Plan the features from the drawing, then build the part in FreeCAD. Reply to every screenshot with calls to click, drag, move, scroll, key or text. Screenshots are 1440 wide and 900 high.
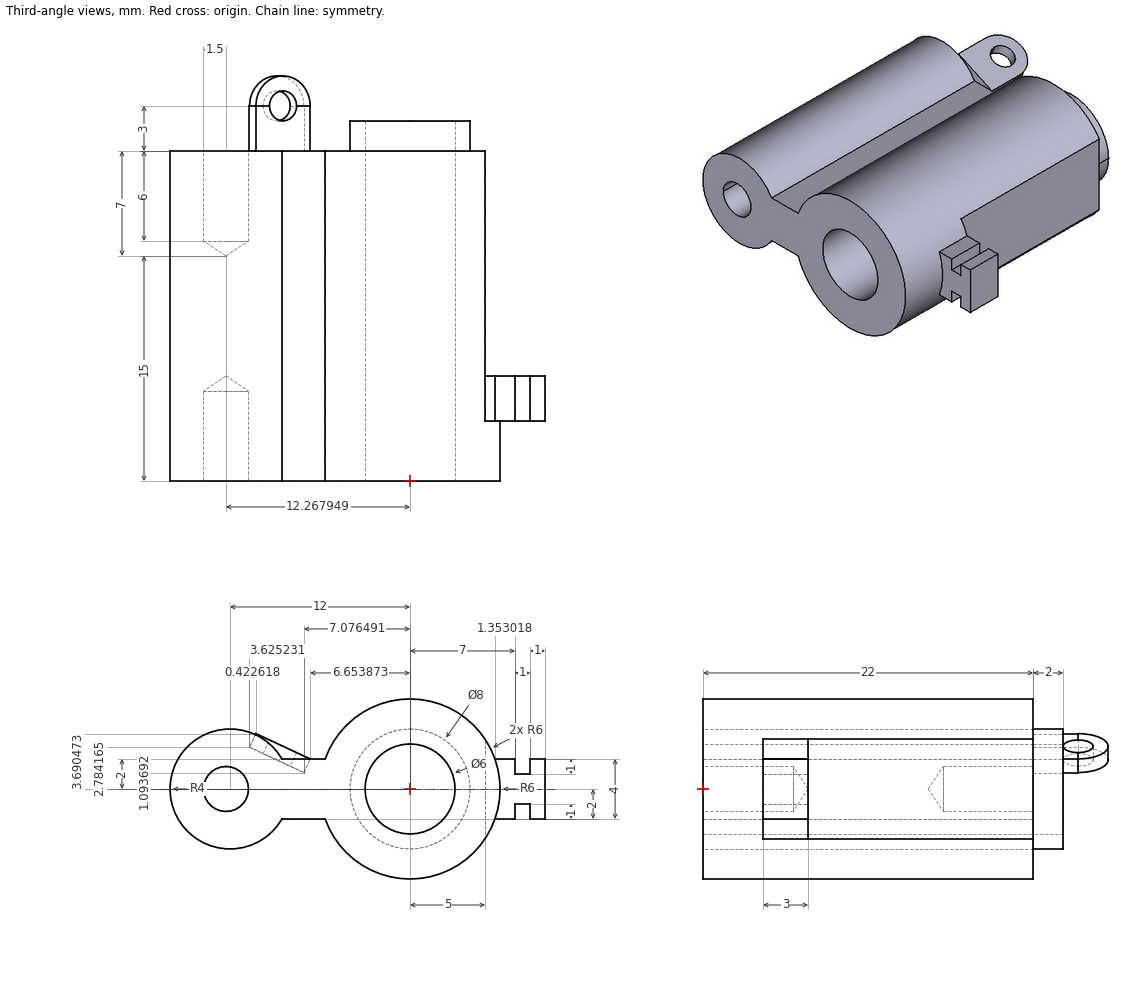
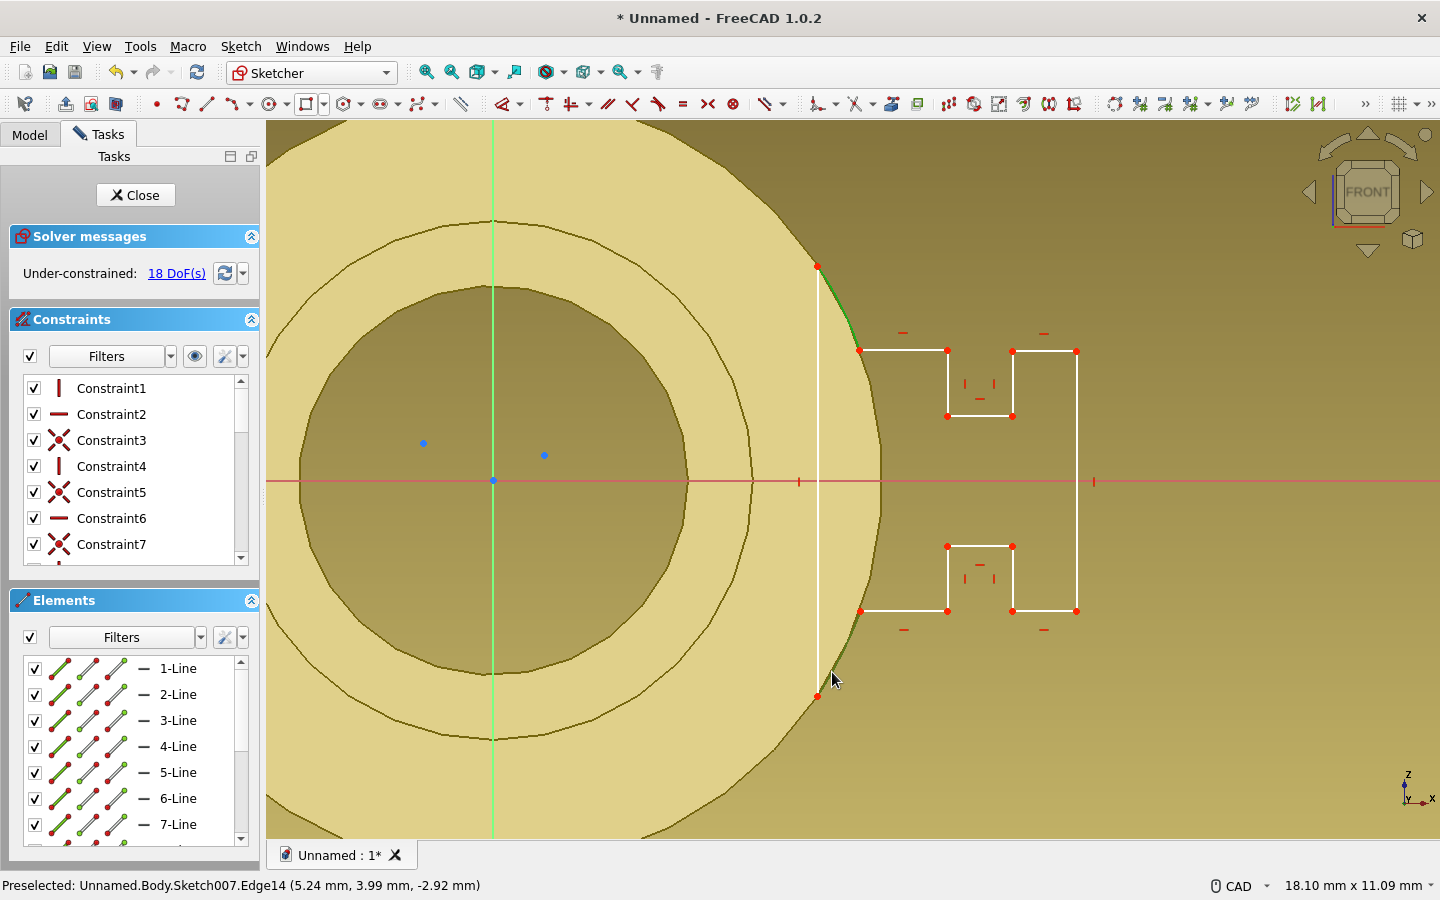
click(546, 104)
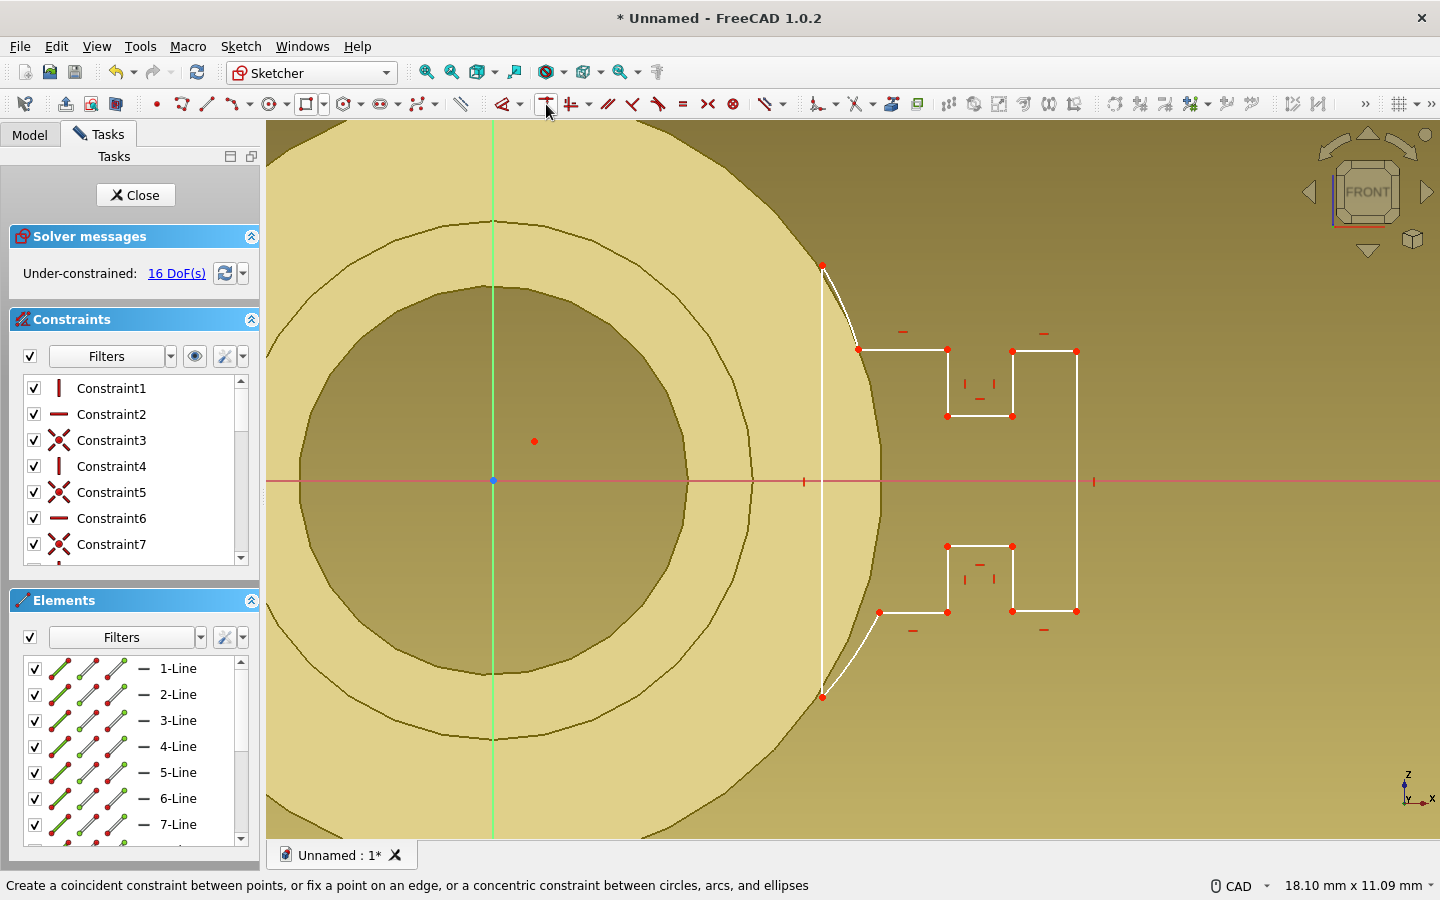
drag(483, 432, 545, 491)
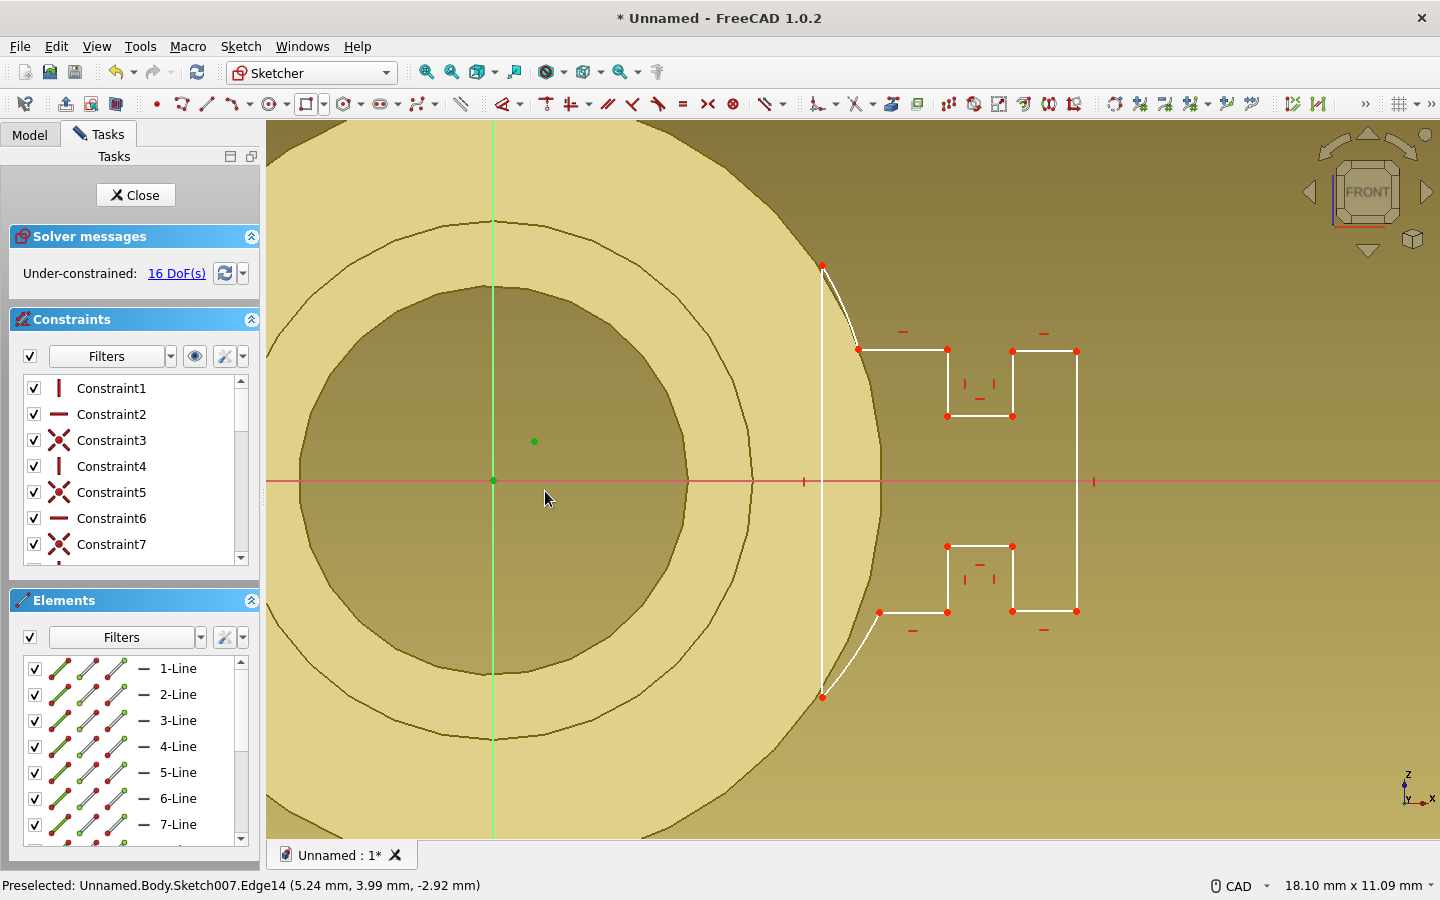
click(546, 104)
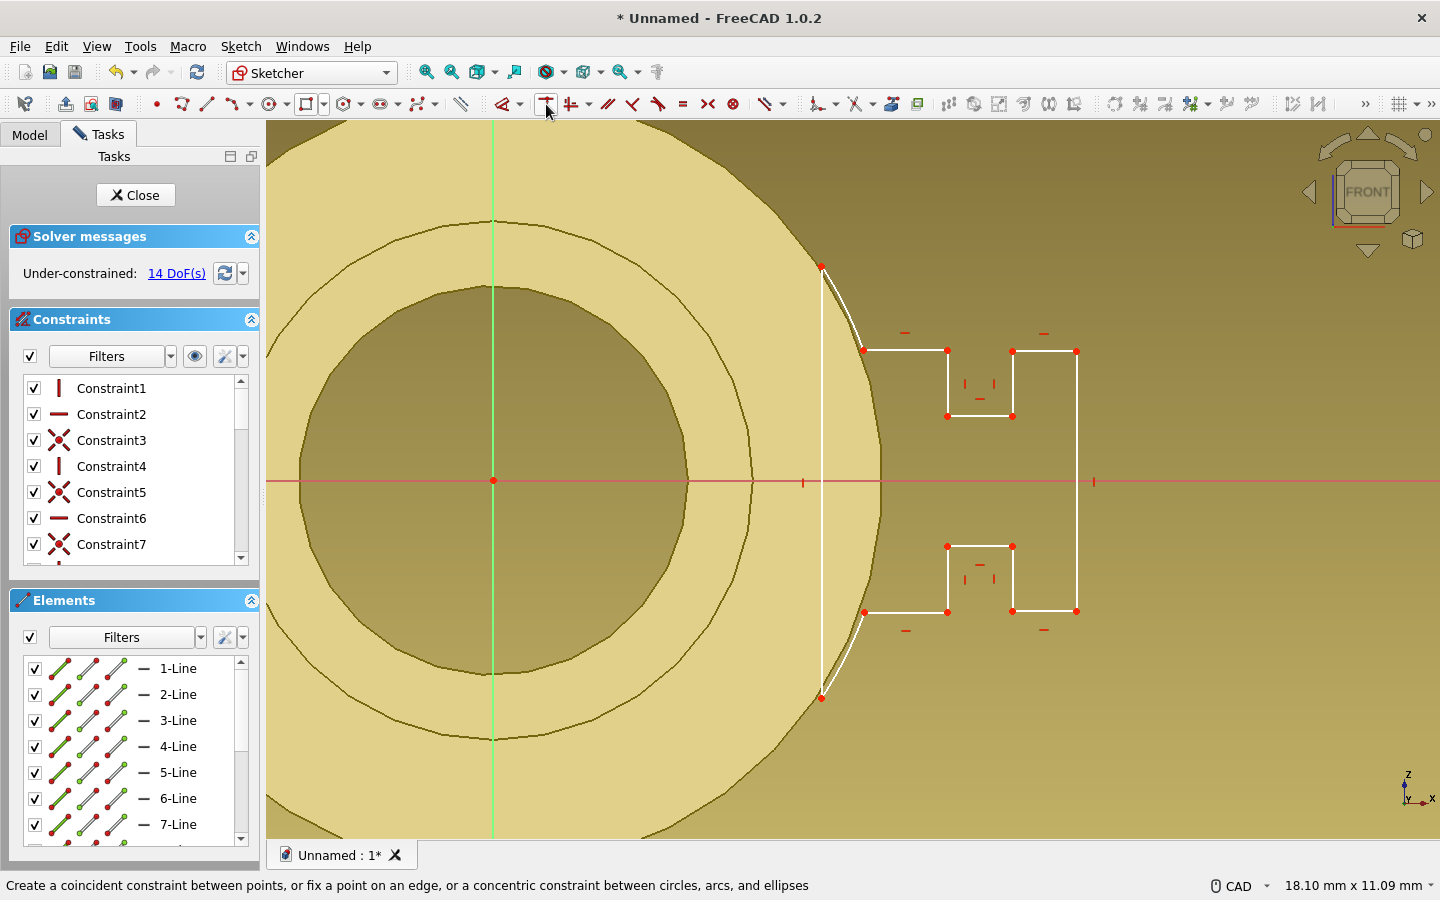
click(853, 324)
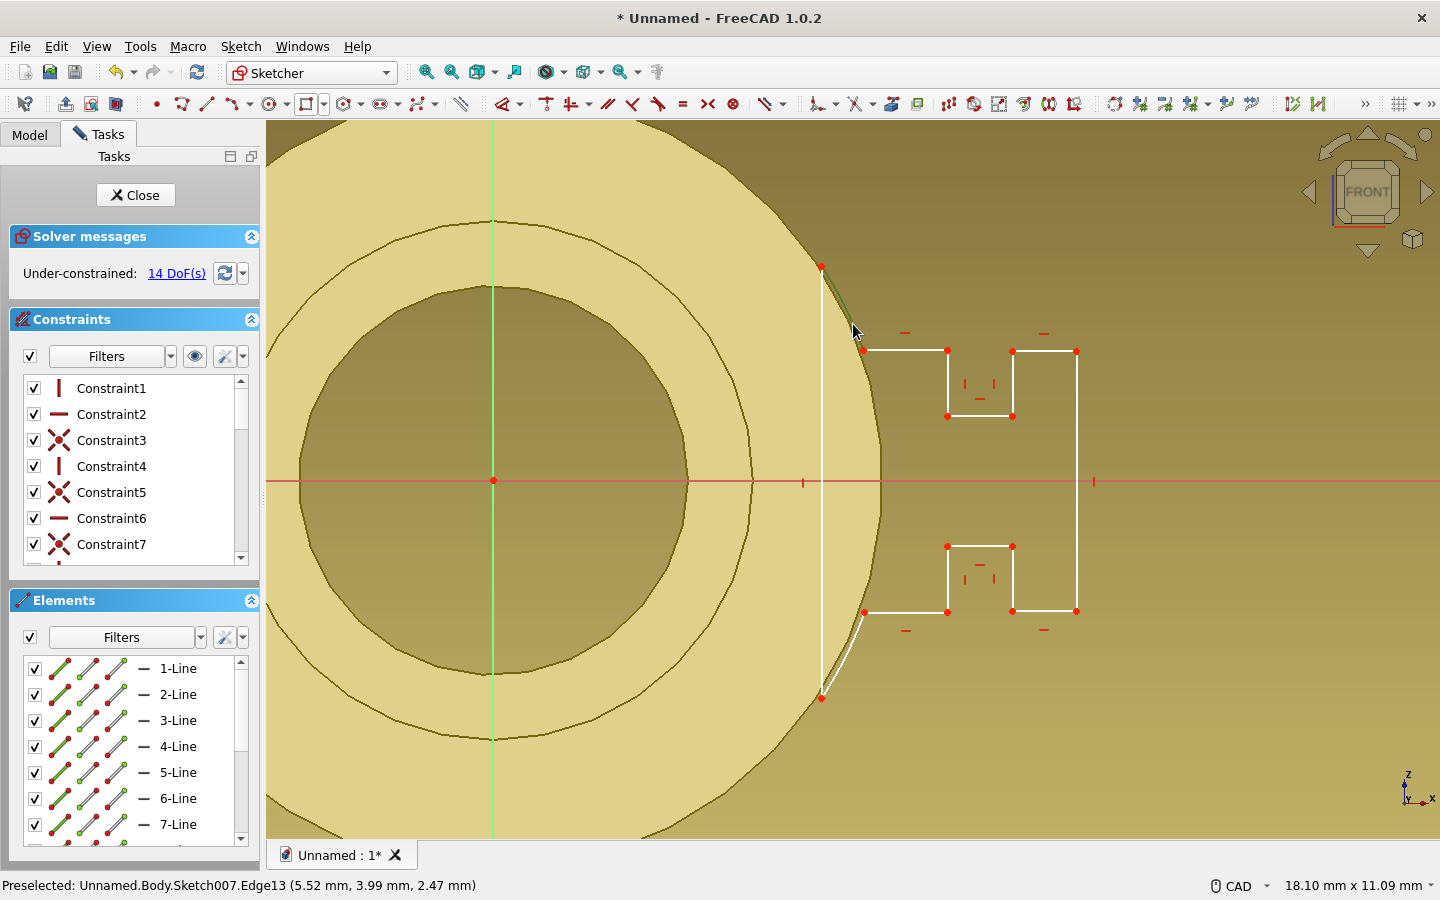
click(837, 674)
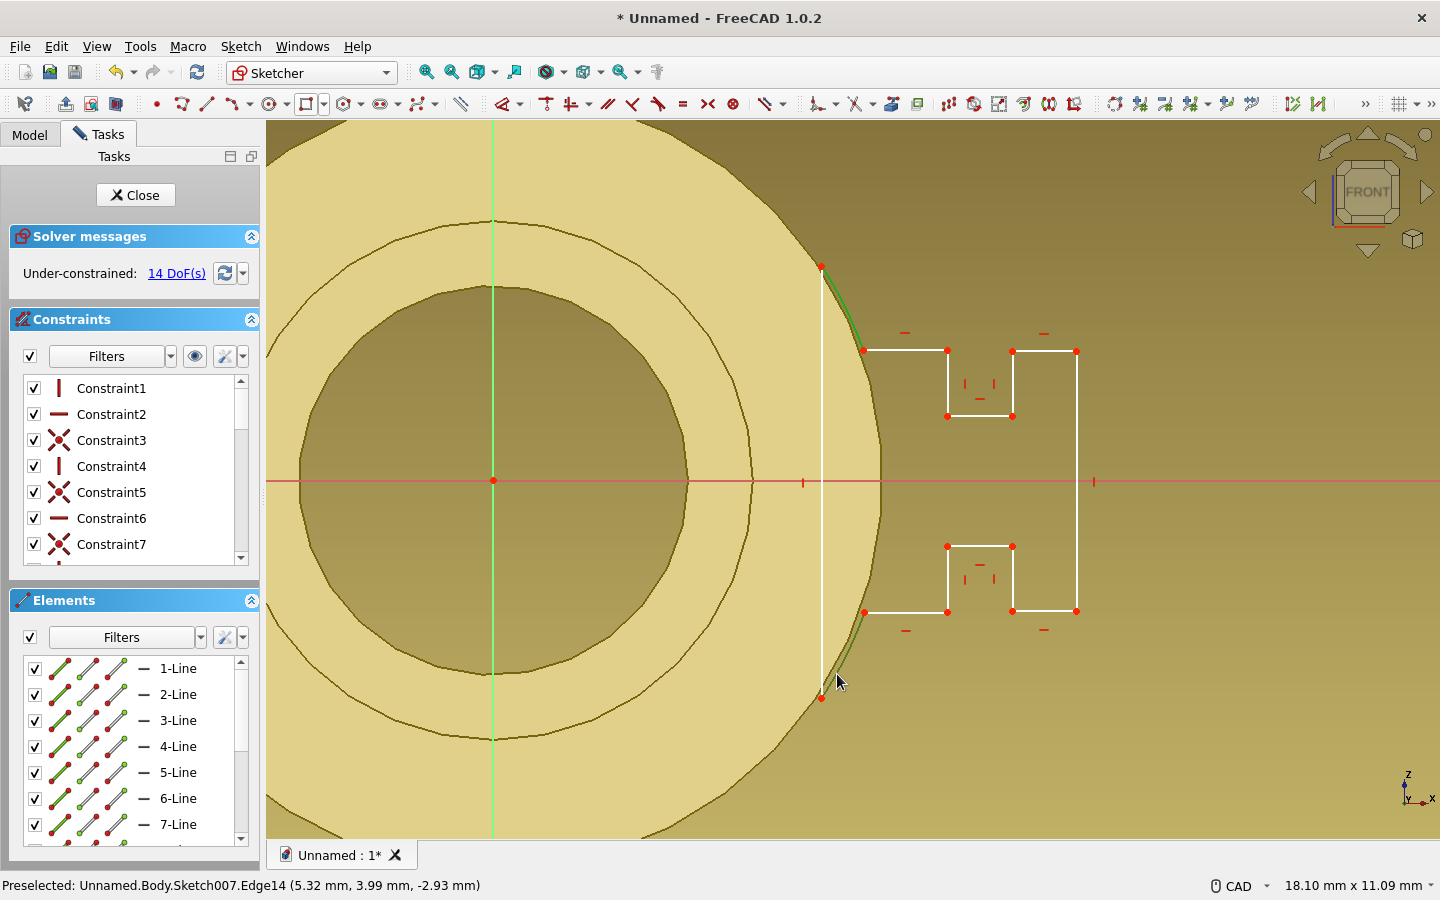
click(683, 104)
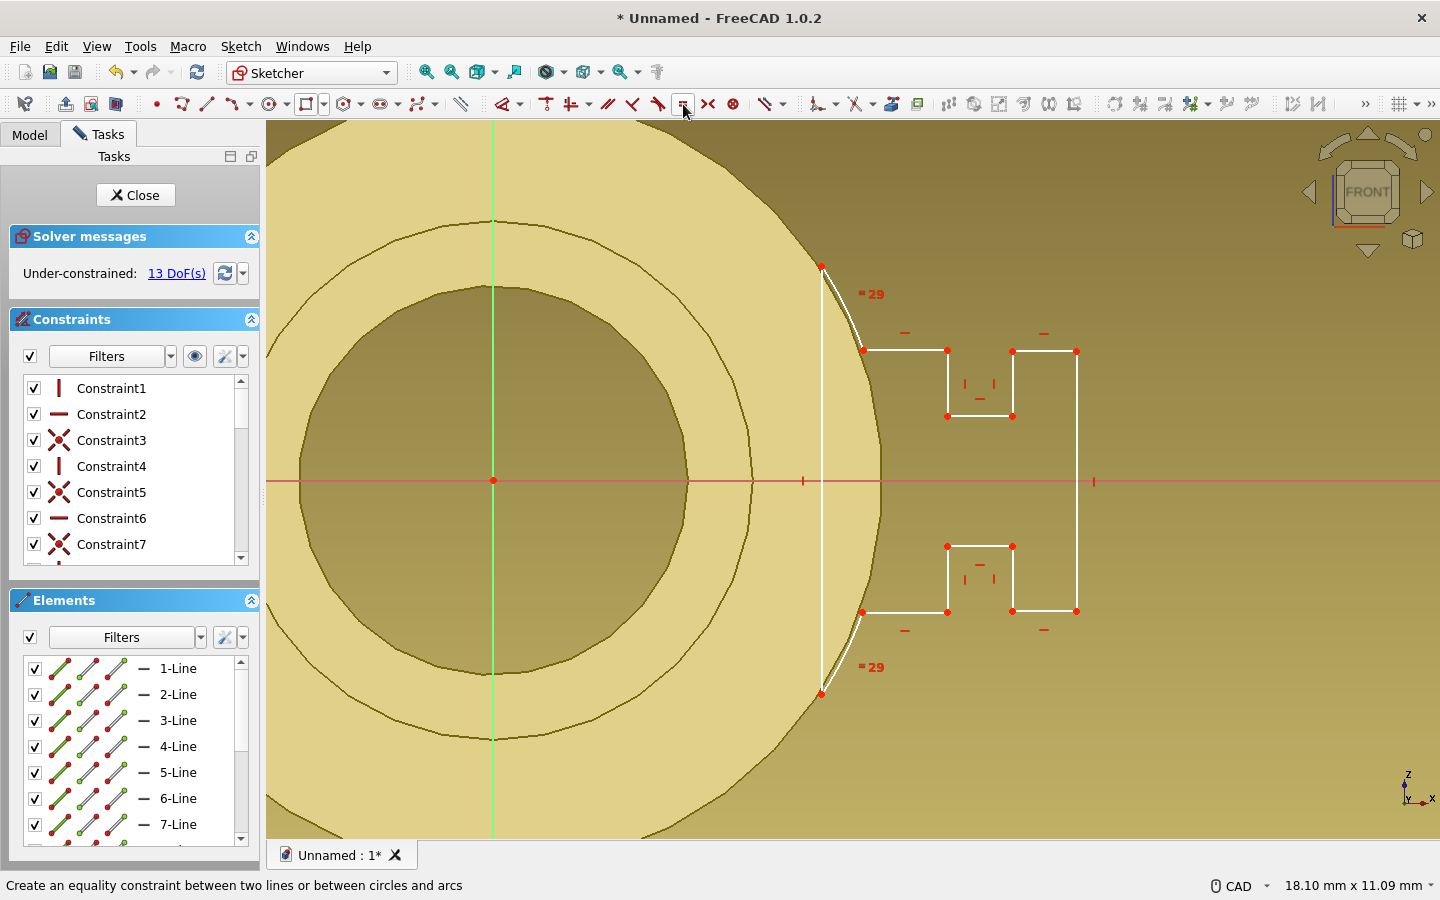
click(1013, 351)